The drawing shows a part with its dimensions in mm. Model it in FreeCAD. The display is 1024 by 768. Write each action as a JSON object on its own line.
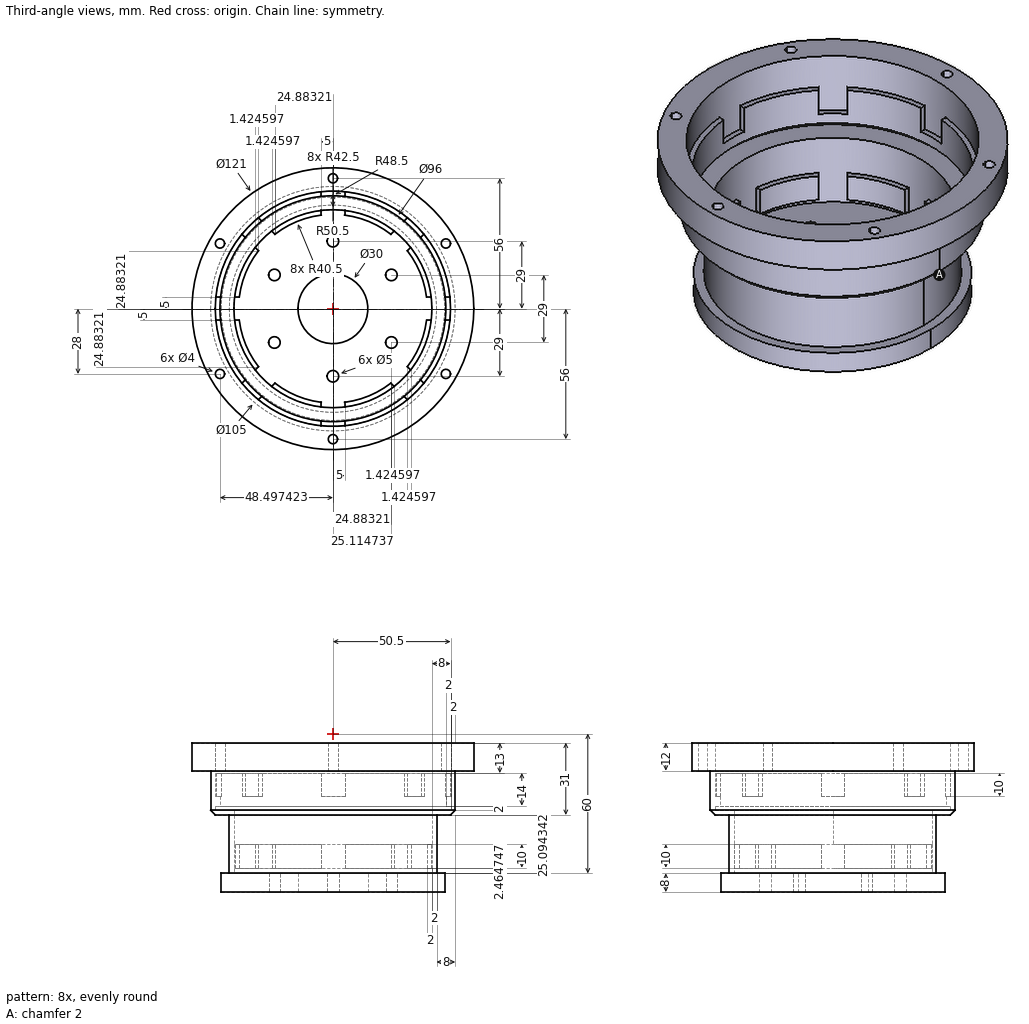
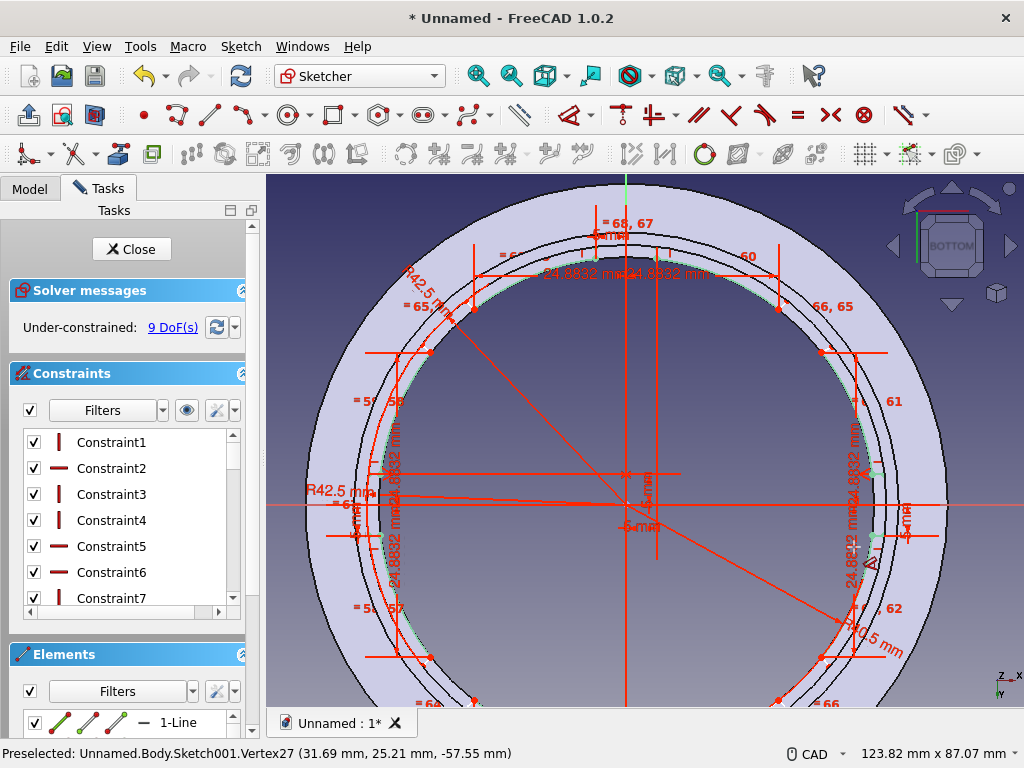
{"action": "scroll", "coordinate": [475, 309], "scroll_direction": "down", "scroll_amount": 2}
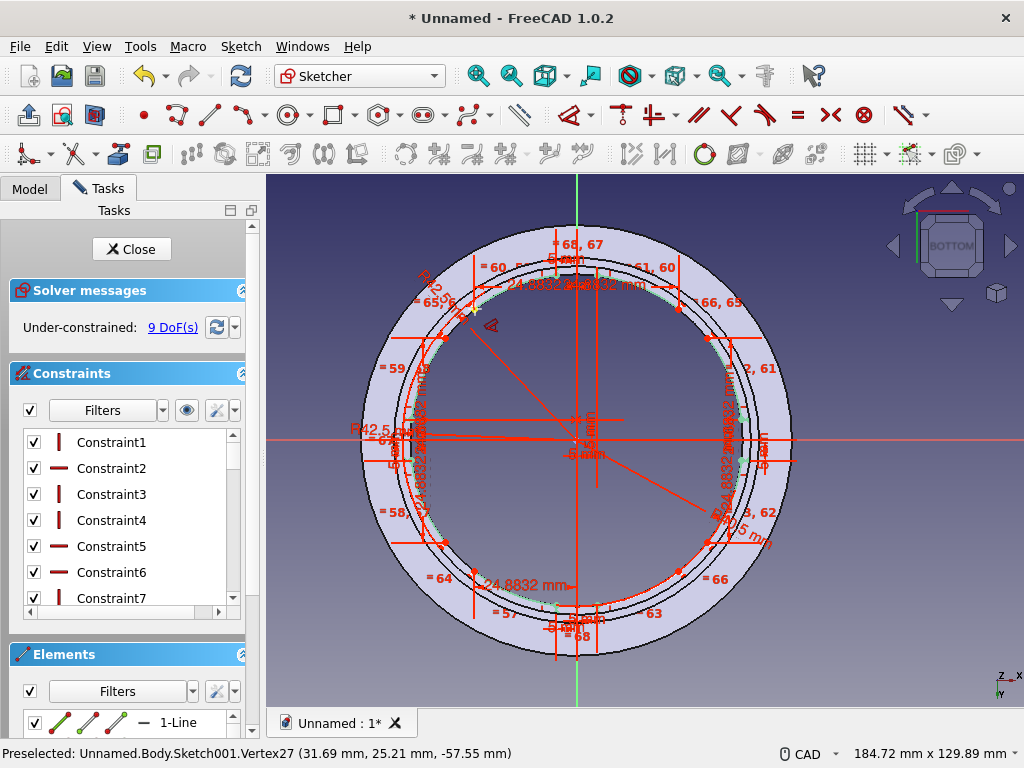
{"action": "scroll", "coordinate": [679, 572], "scroll_direction": "up", "scroll_amount": 2}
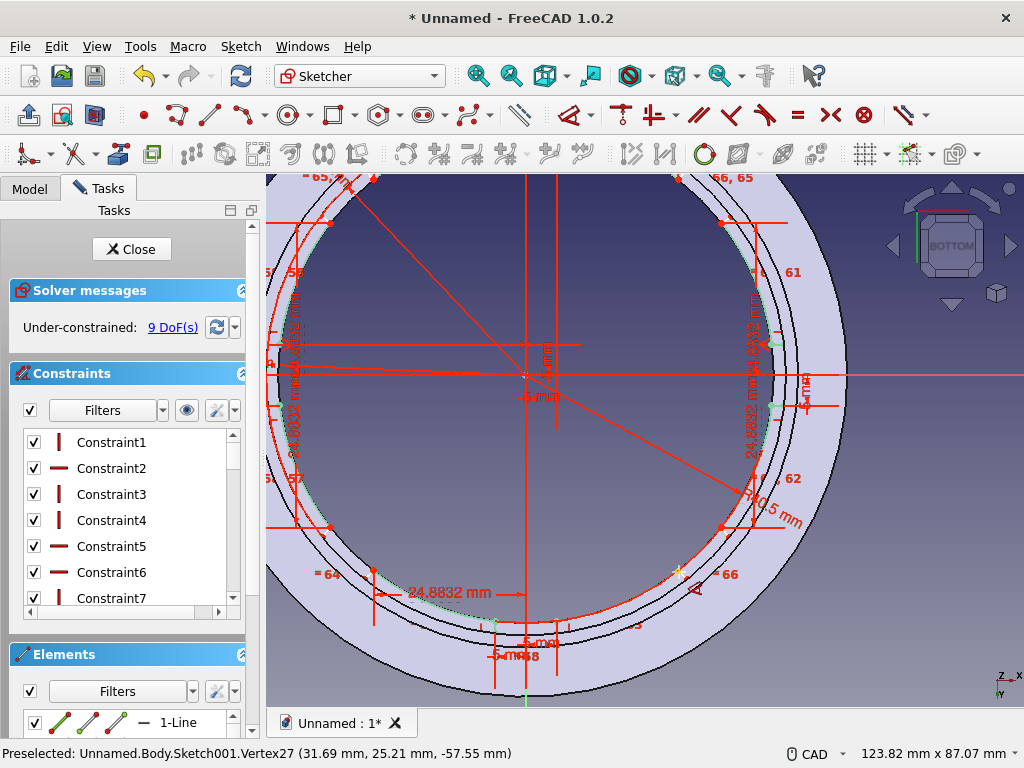
{"action": "left_click", "coordinate": [678, 571]}
{"action": "left_click", "coordinate": [567, 605]}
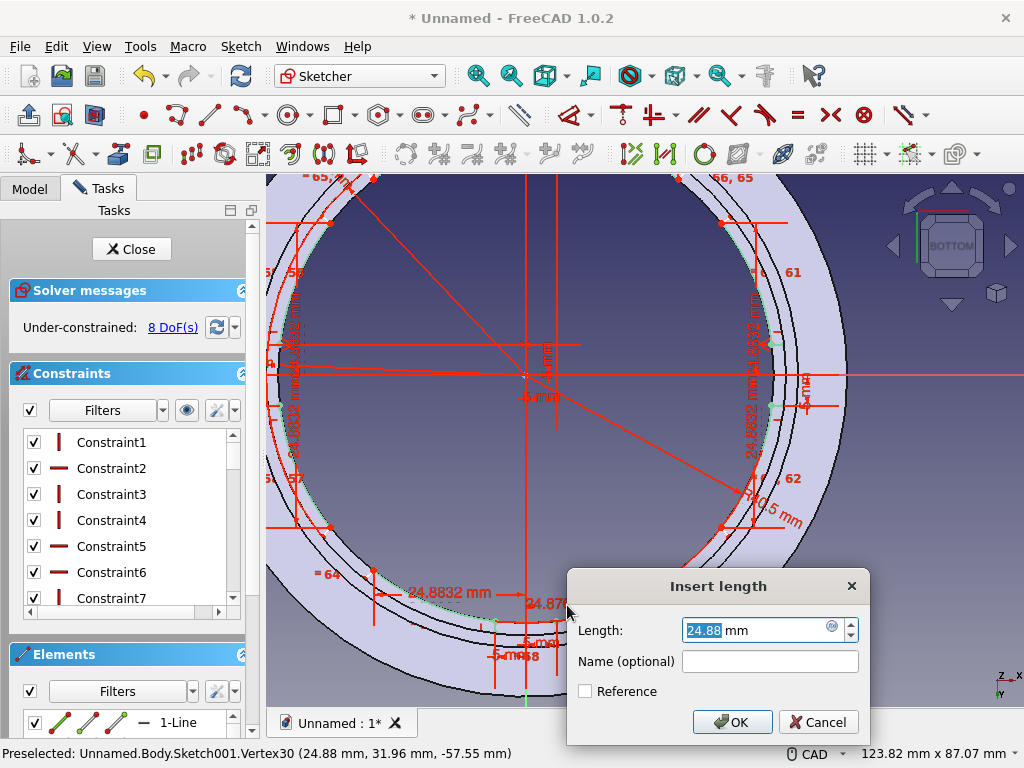
{"action": "type", "text": "24.88321"}
{"action": "key", "text": "Return"}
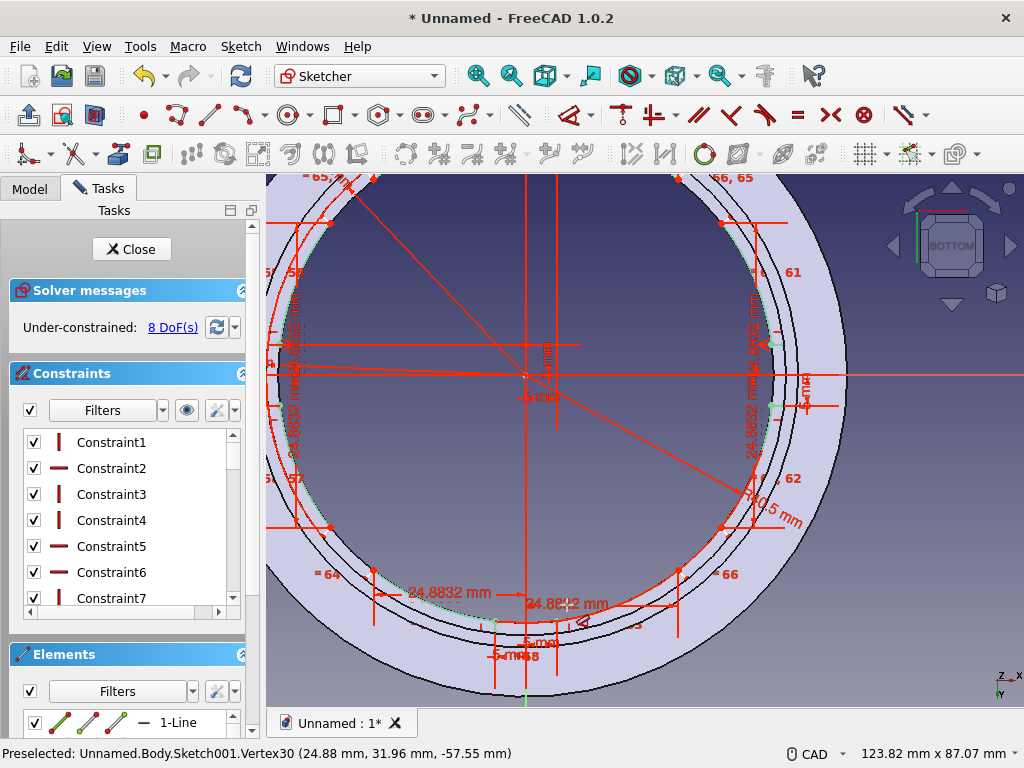
{"action": "scroll", "coordinate": [369, 575], "scroll_direction": "up", "scroll_amount": 8}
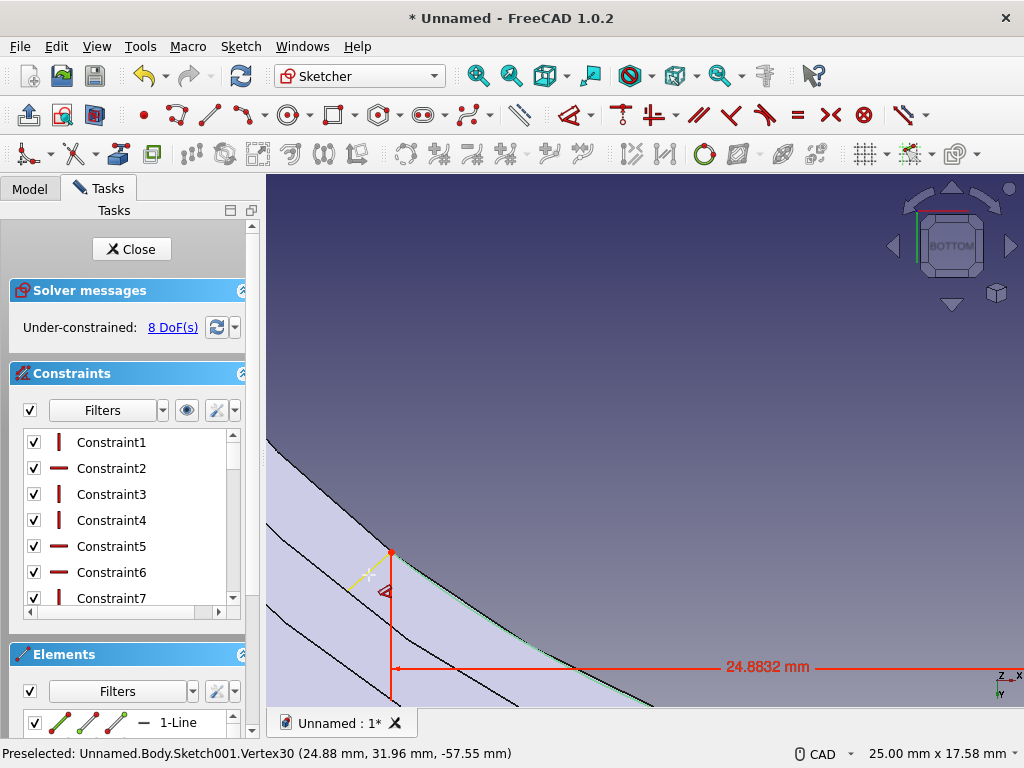
{"action": "left_click", "coordinate": [368, 573]}
{"action": "left_click", "coordinate": [368, 627]}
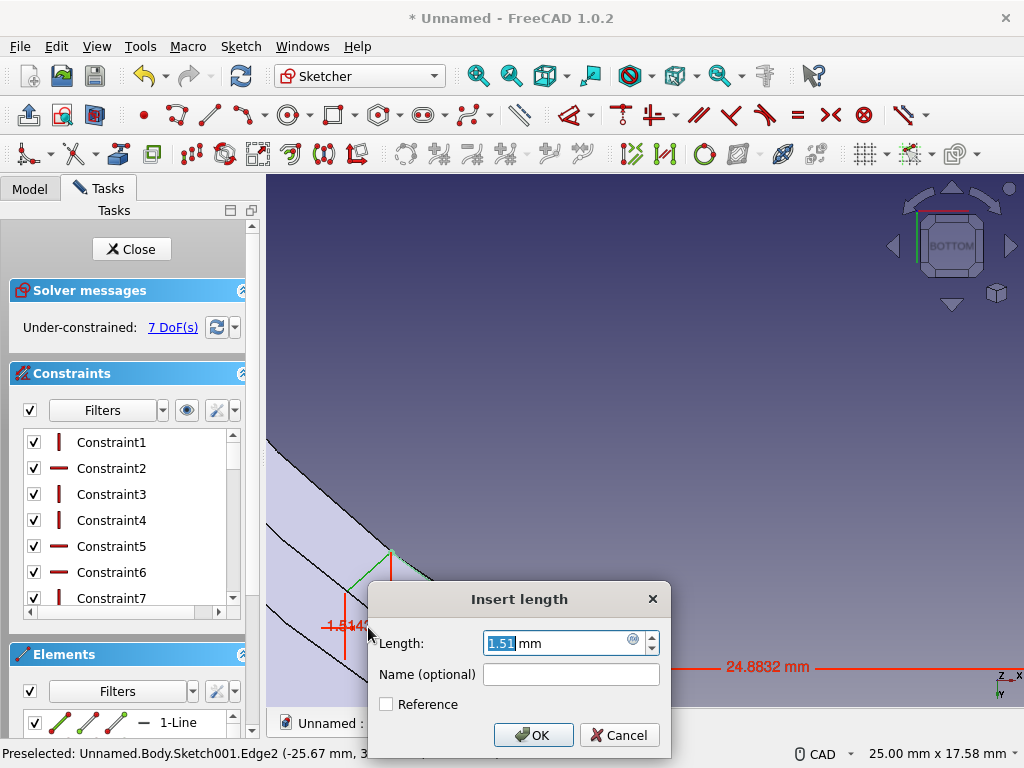
{"action": "type", "text": "1.424597"}
{"action": "key", "text": "Return"}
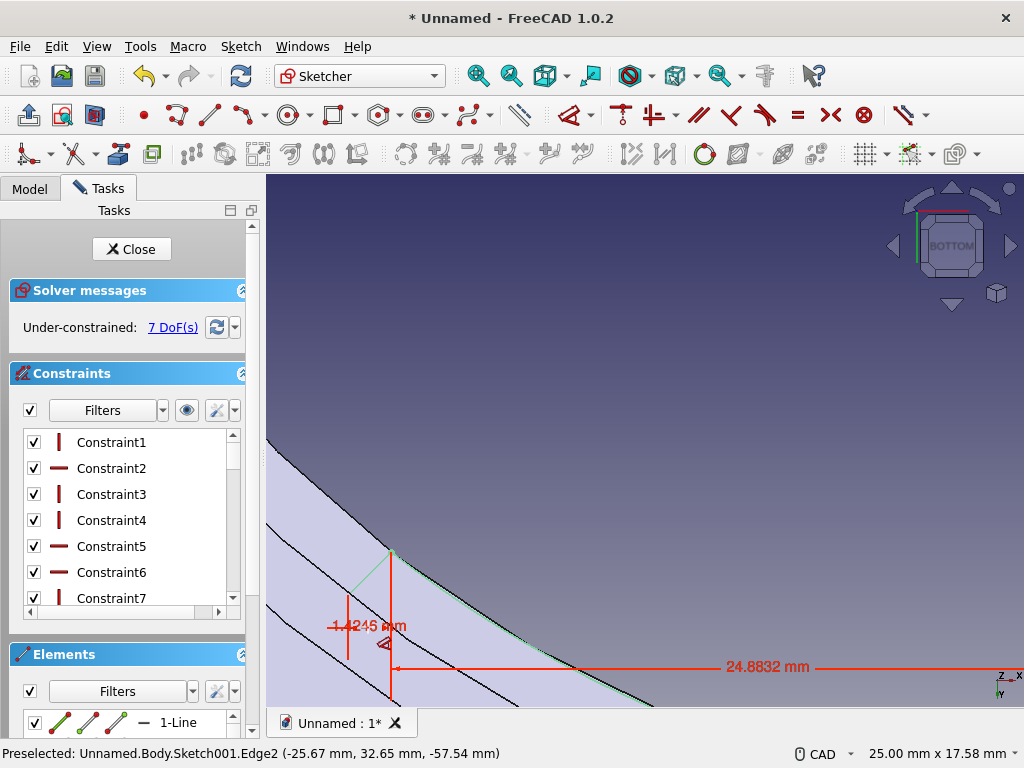
{"action": "scroll", "coordinate": [487, 575], "scroll_direction": "down", "scroll_amount": 10}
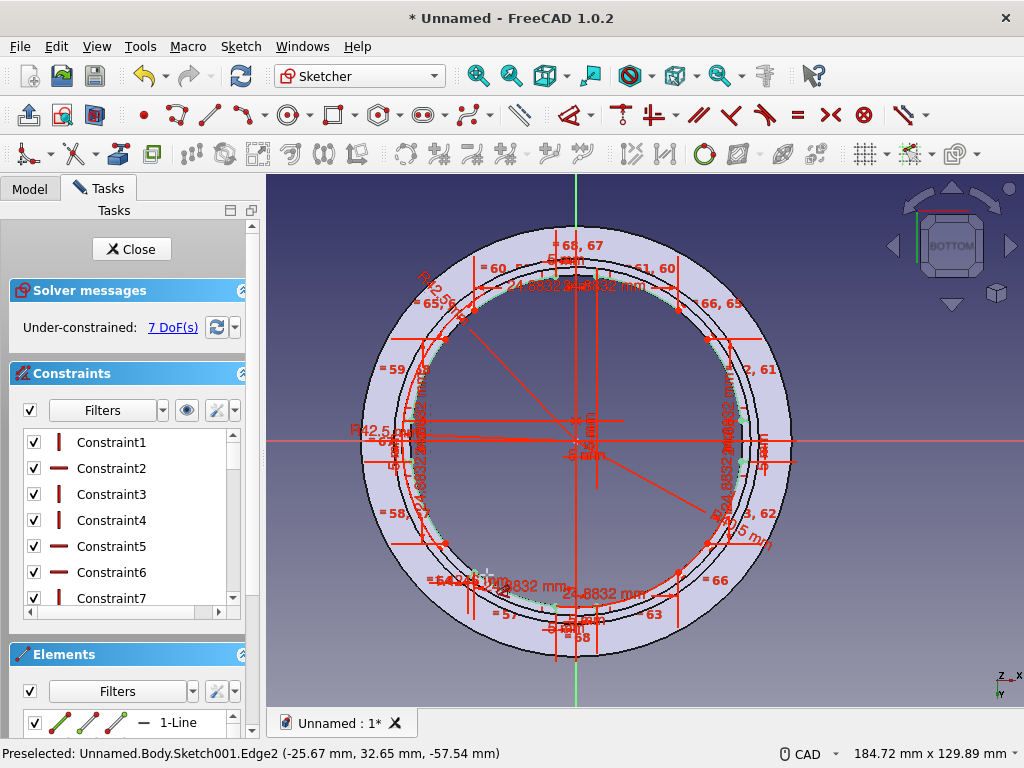
{"action": "scroll", "coordinate": [441, 548], "scroll_direction": "up", "scroll_amount": 10}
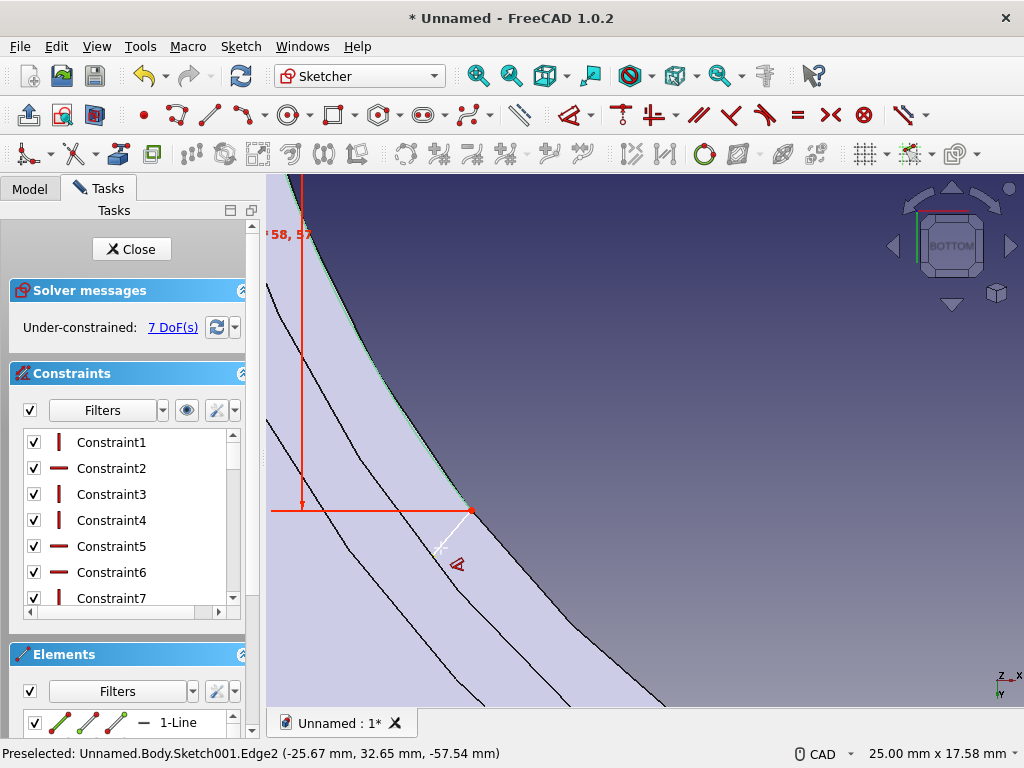
{"action": "left_click", "coordinate": [443, 544]}
{"action": "left_click", "coordinate": [442, 592]}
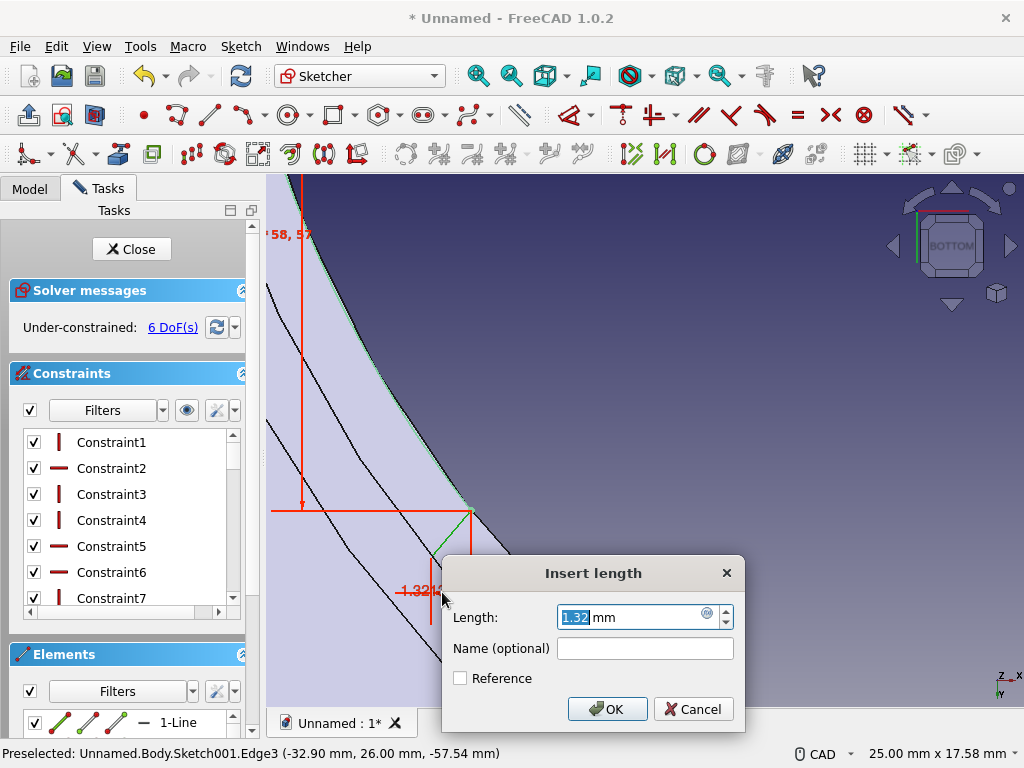
{"action": "type", "text": "1.424597"}
{"action": "key", "text": "Return"}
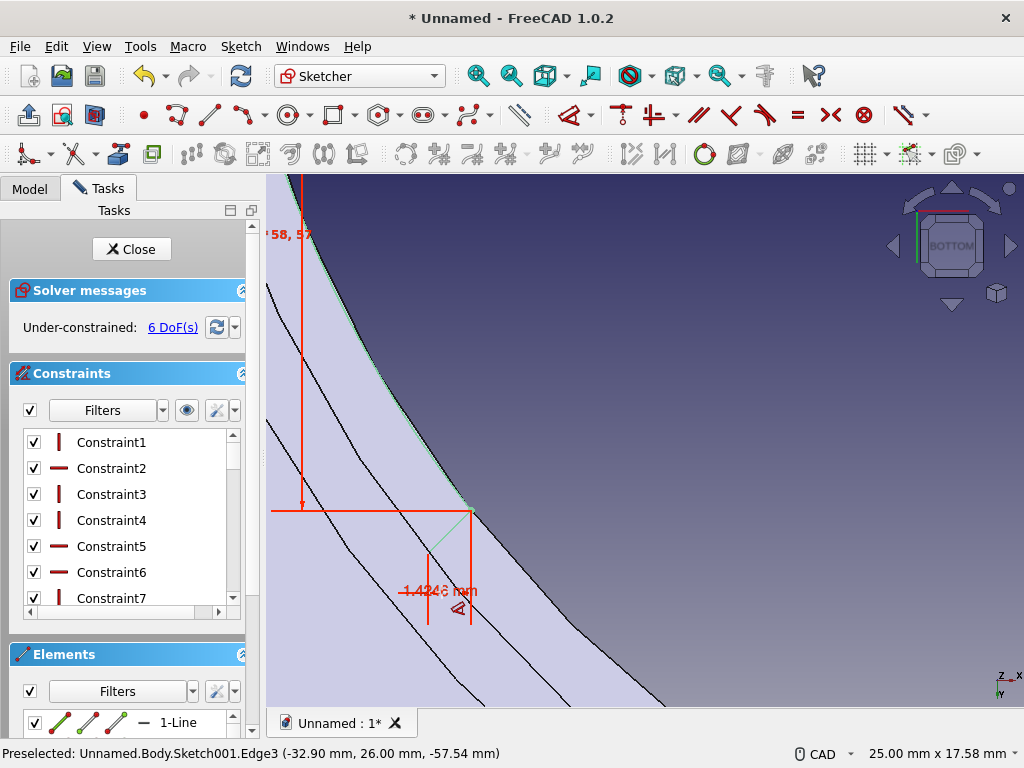
{"action": "scroll", "coordinate": [441, 548], "scroll_direction": "down", "scroll_amount": 10}